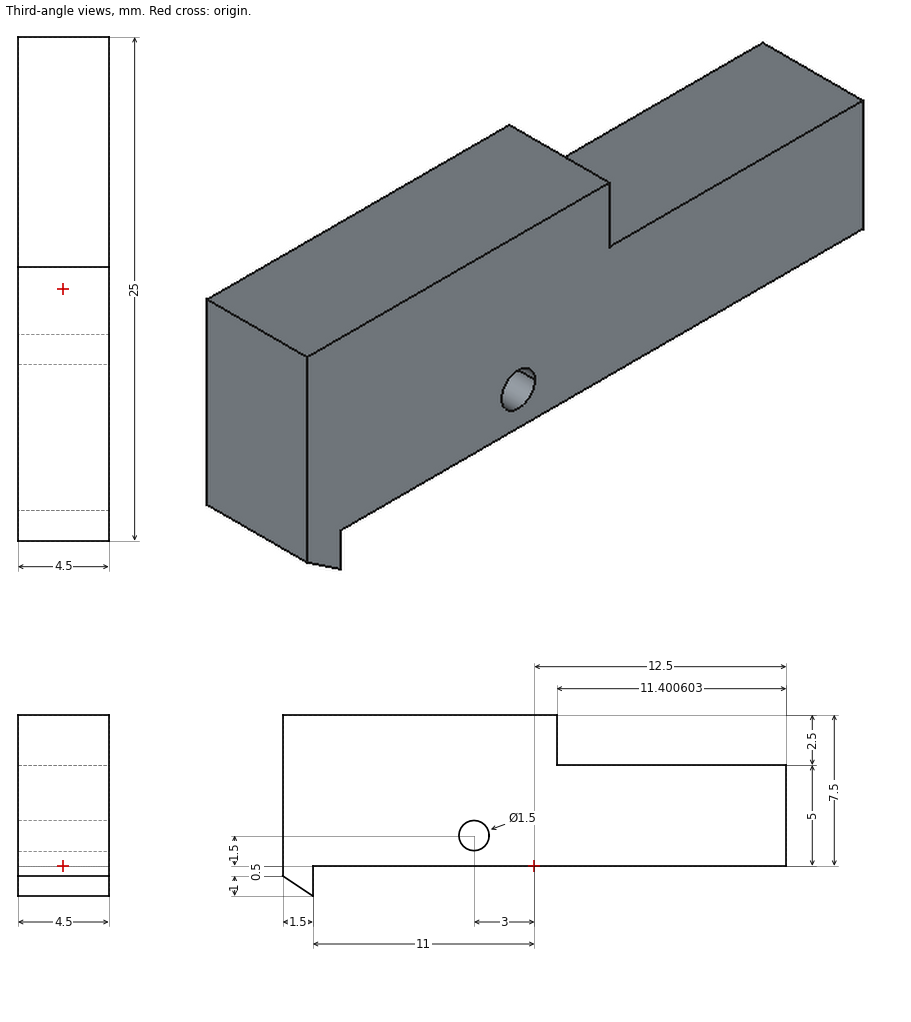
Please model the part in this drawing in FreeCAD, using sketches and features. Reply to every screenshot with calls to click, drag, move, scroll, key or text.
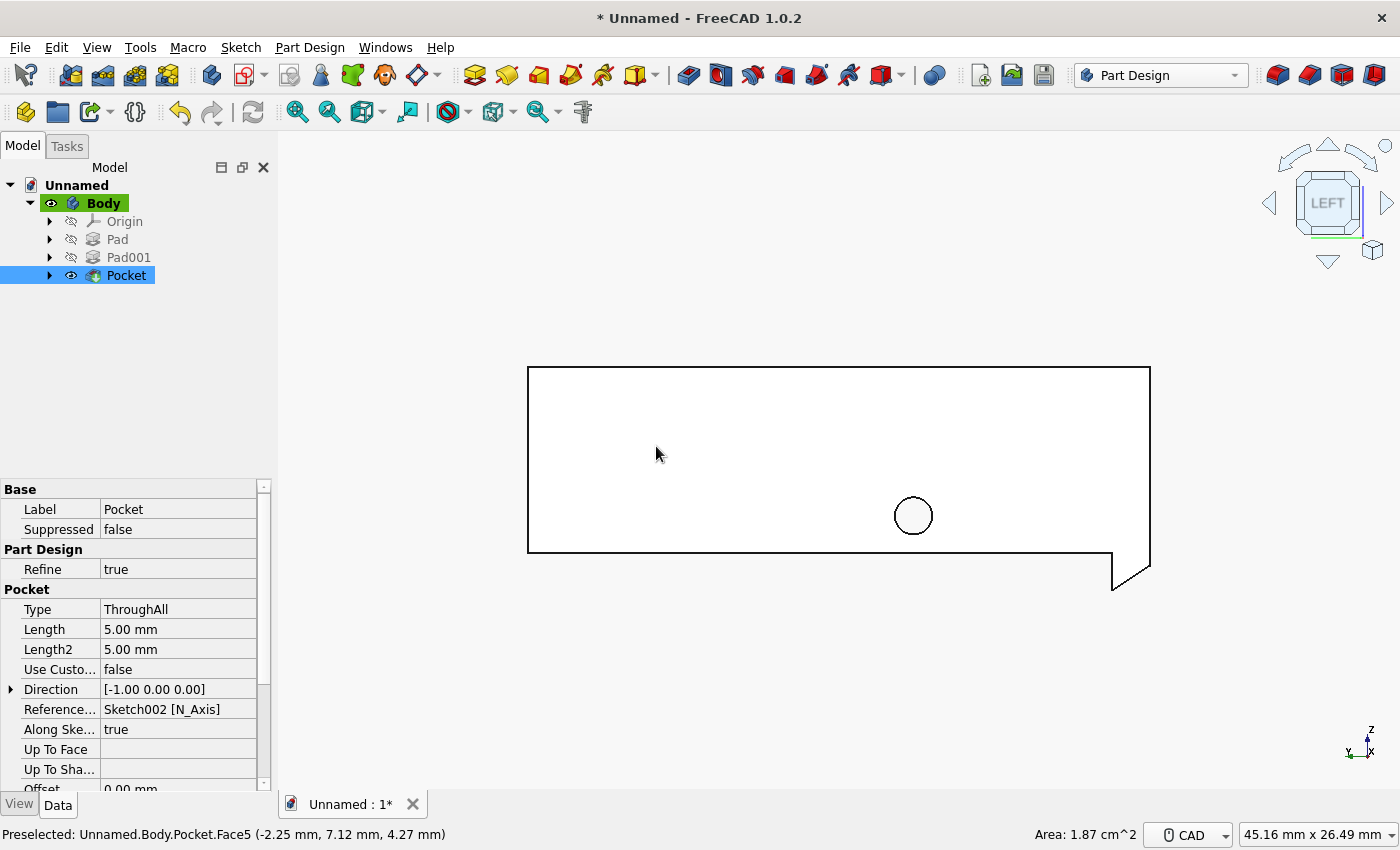
click(244, 76)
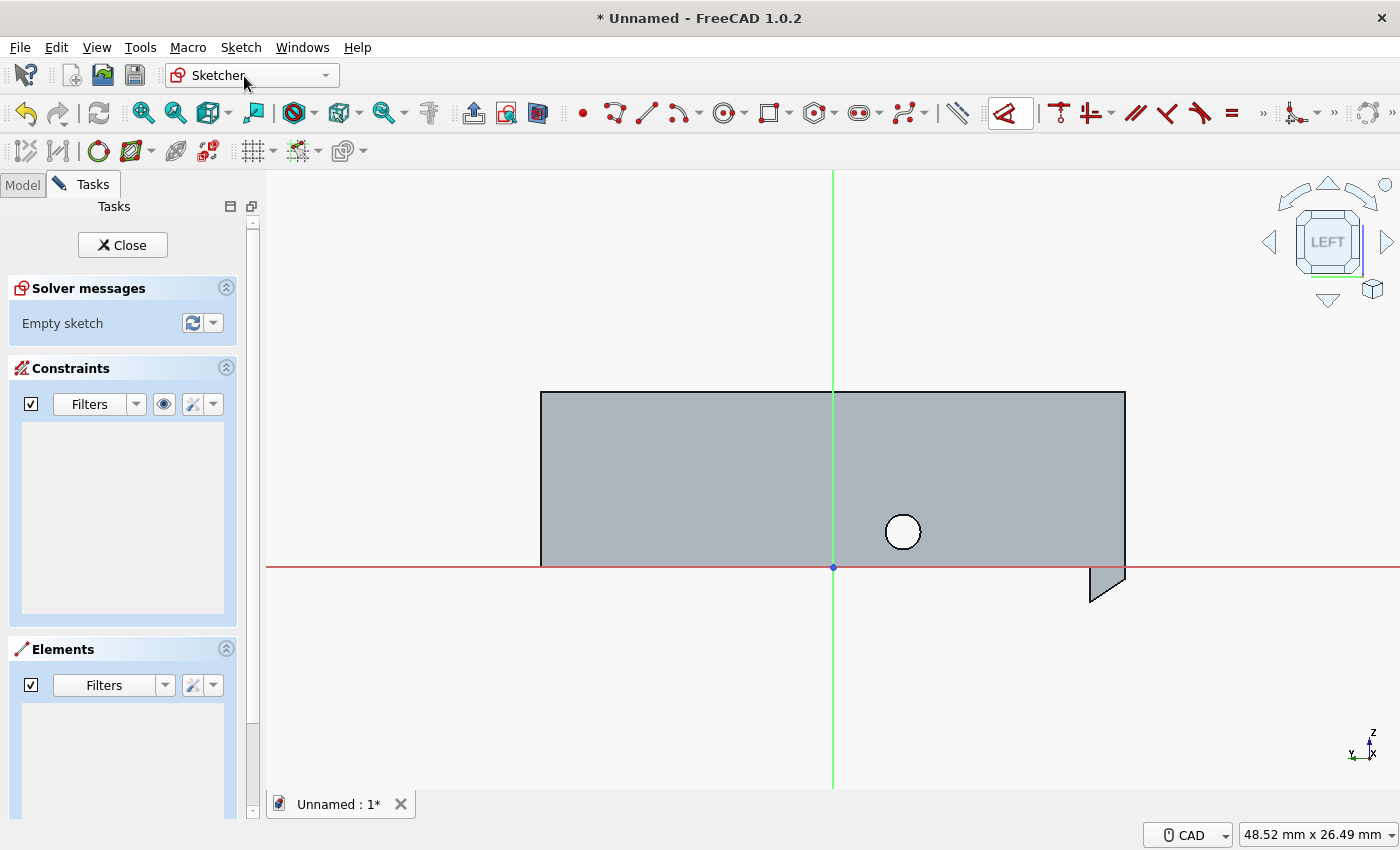
scroll(624, 479, up, 4)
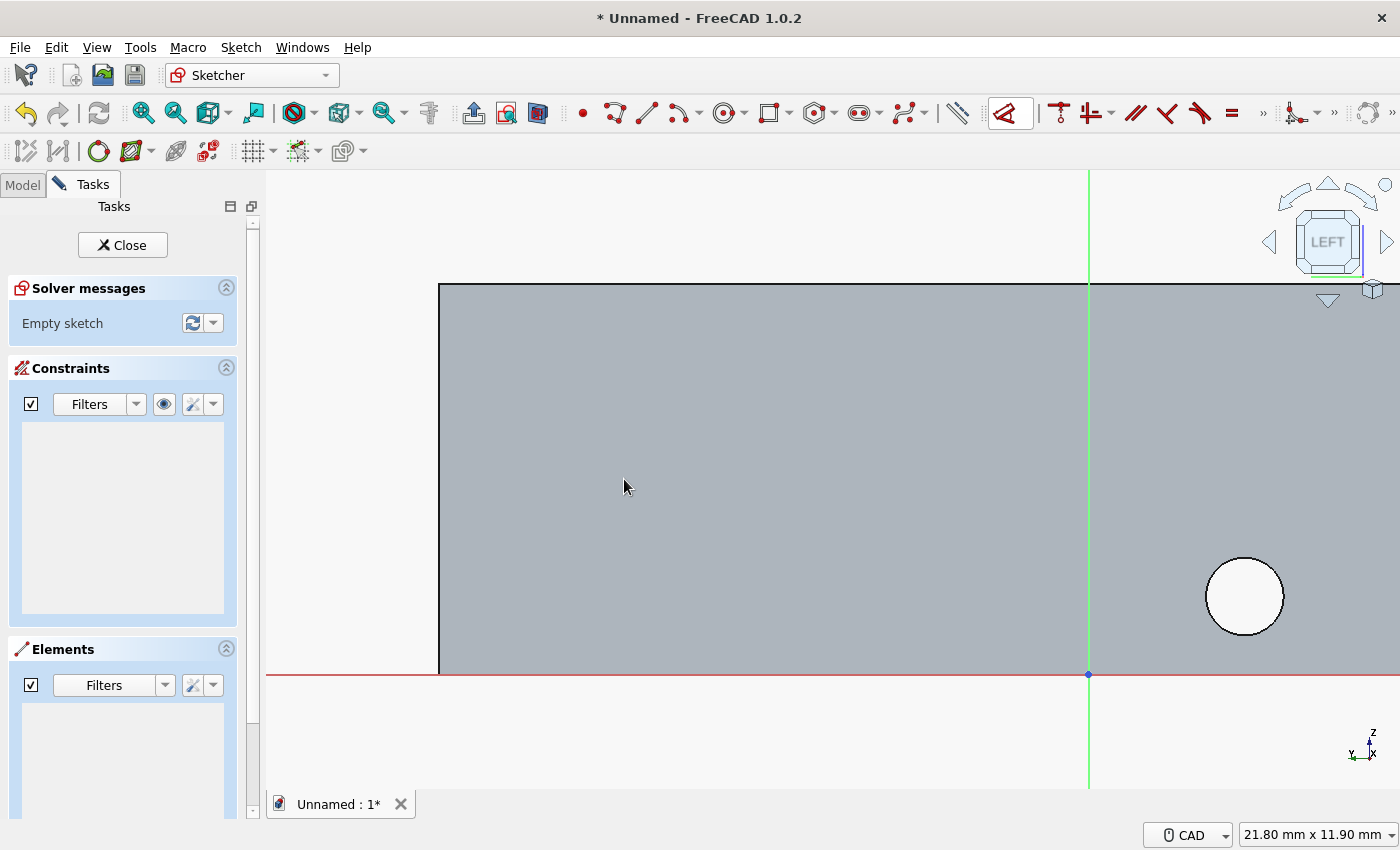
key(g)
key(r)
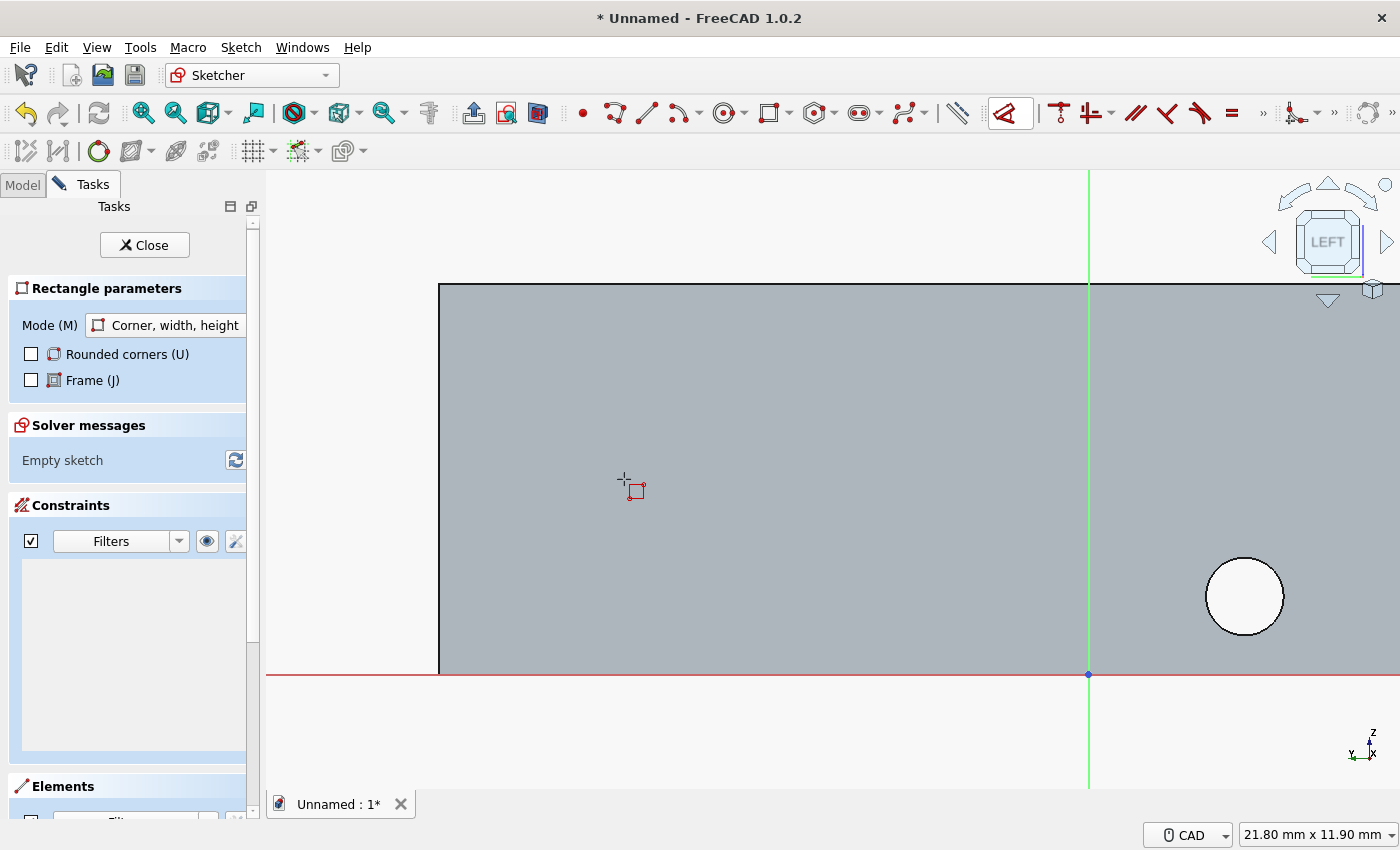
click(439, 284)
move(1032, 414)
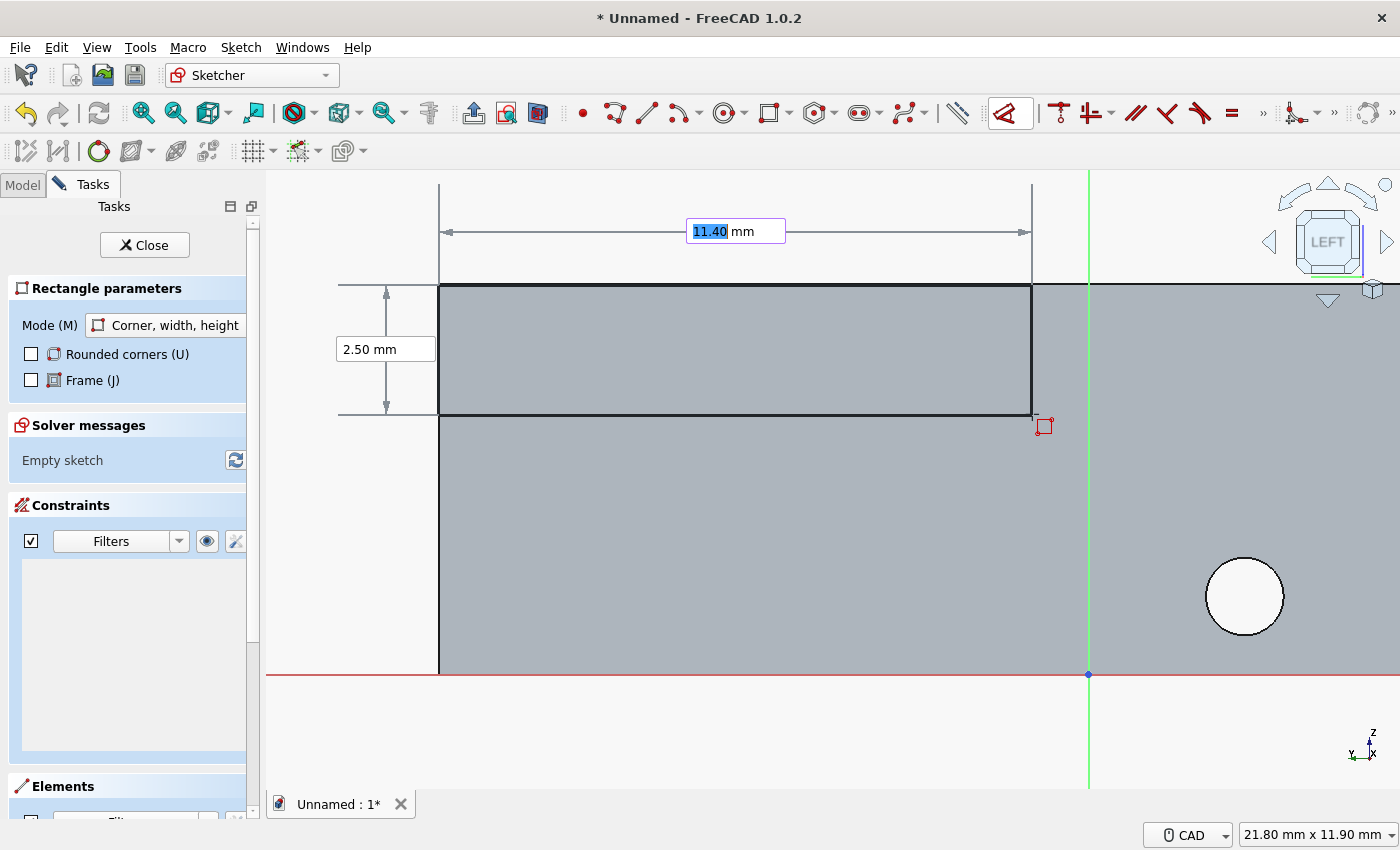
text(11.400603)
key(Tab)
text(2.5)
key(Return)
key(Escape)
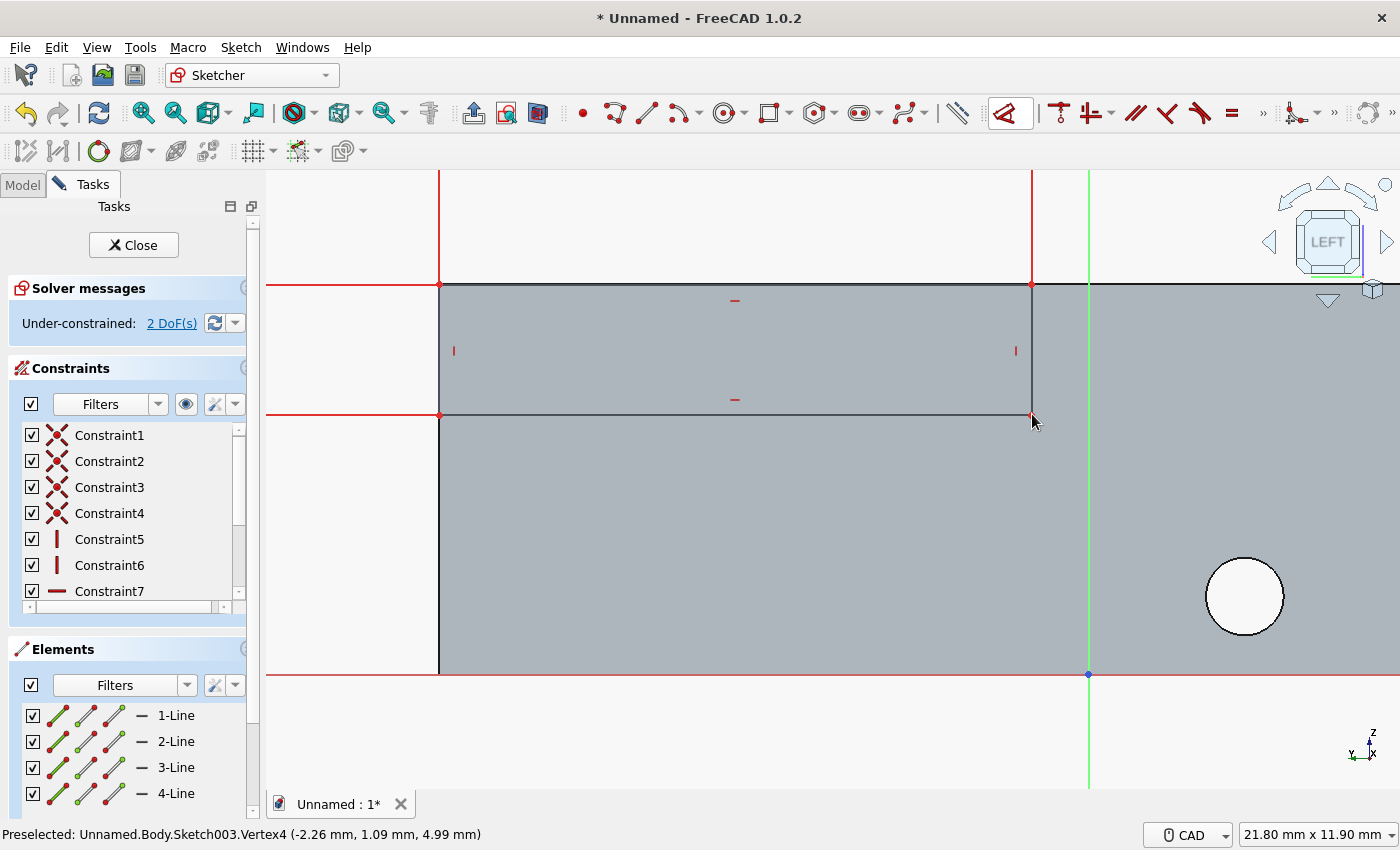
click(439, 415)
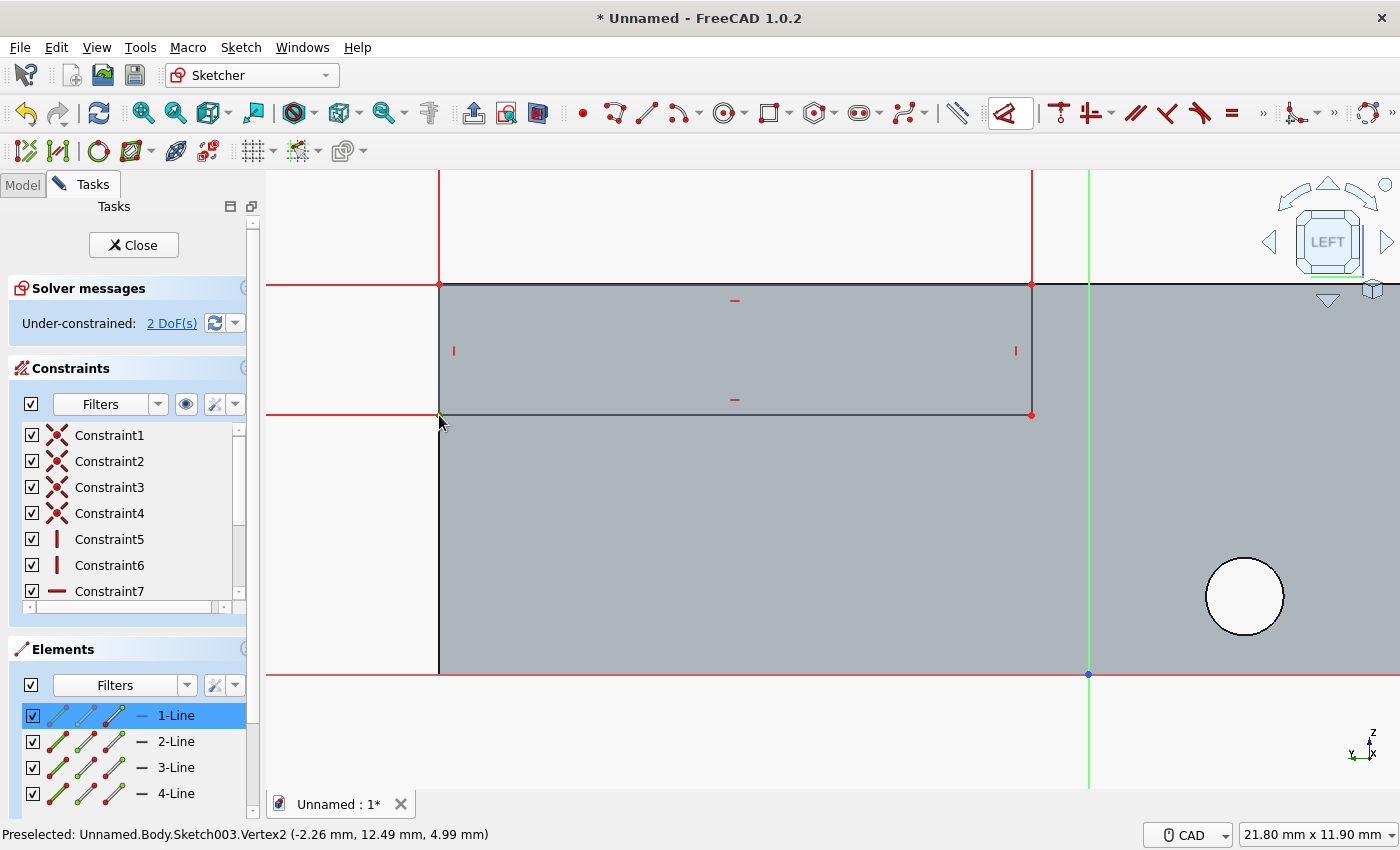
key(i)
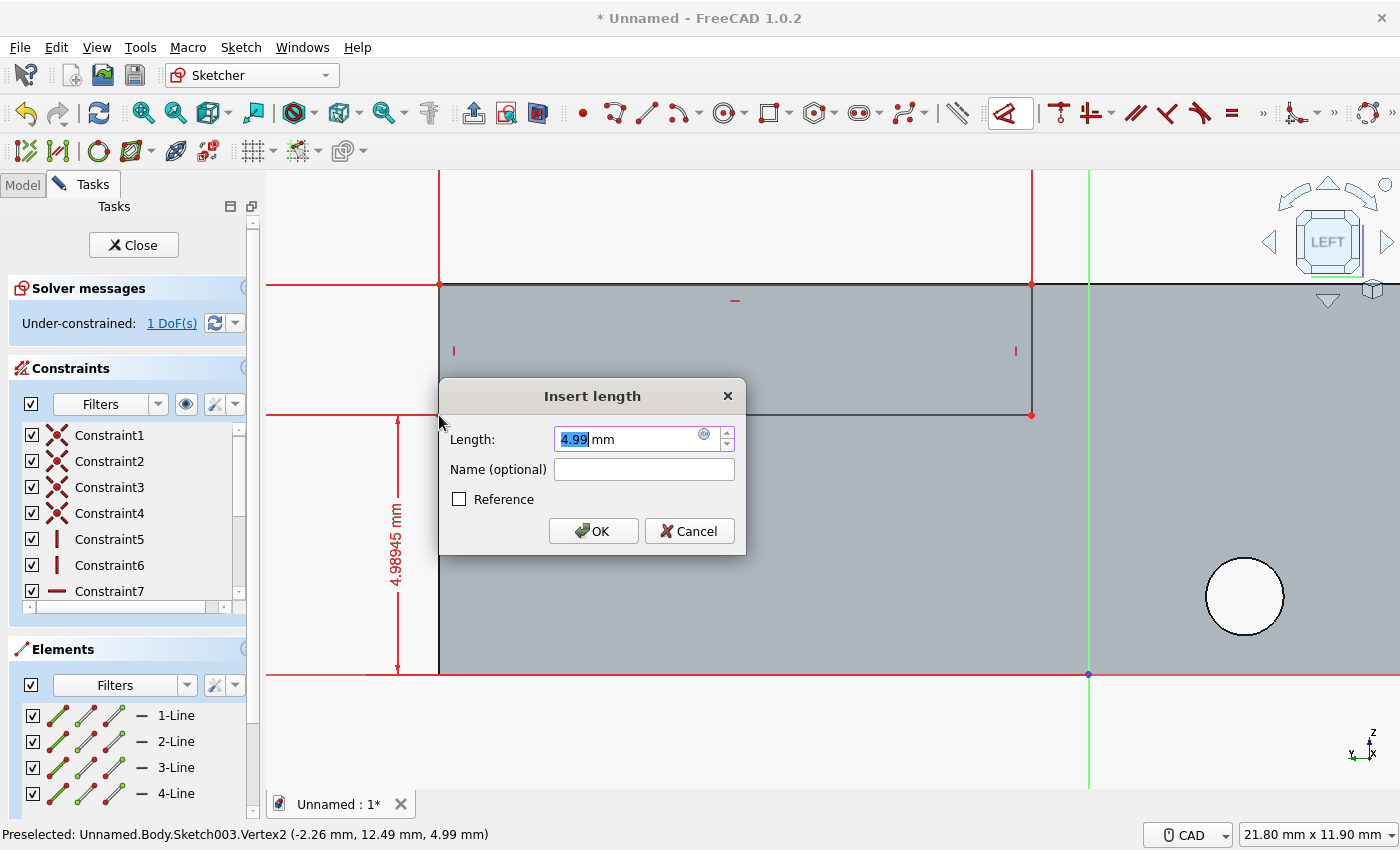
text(5)
key(Return)